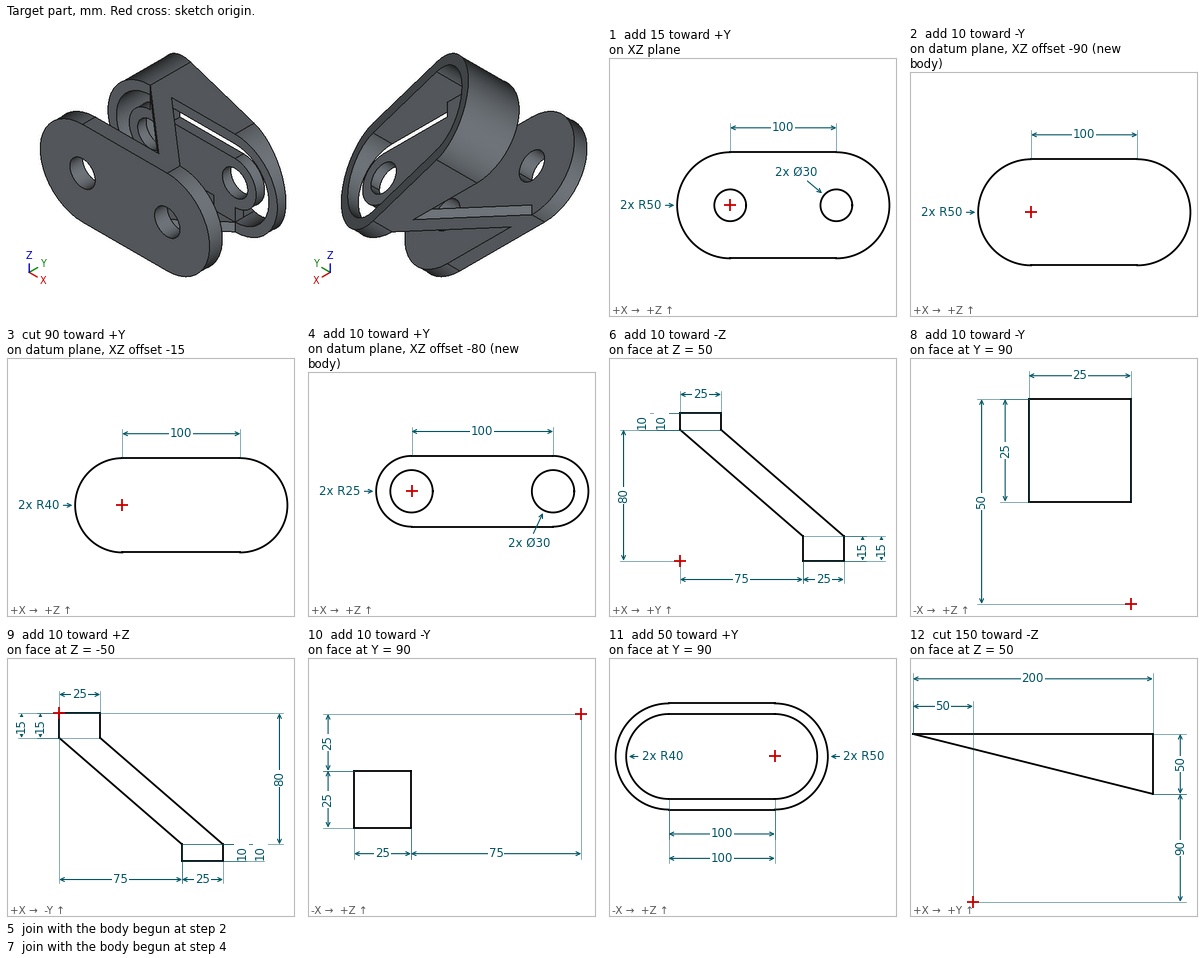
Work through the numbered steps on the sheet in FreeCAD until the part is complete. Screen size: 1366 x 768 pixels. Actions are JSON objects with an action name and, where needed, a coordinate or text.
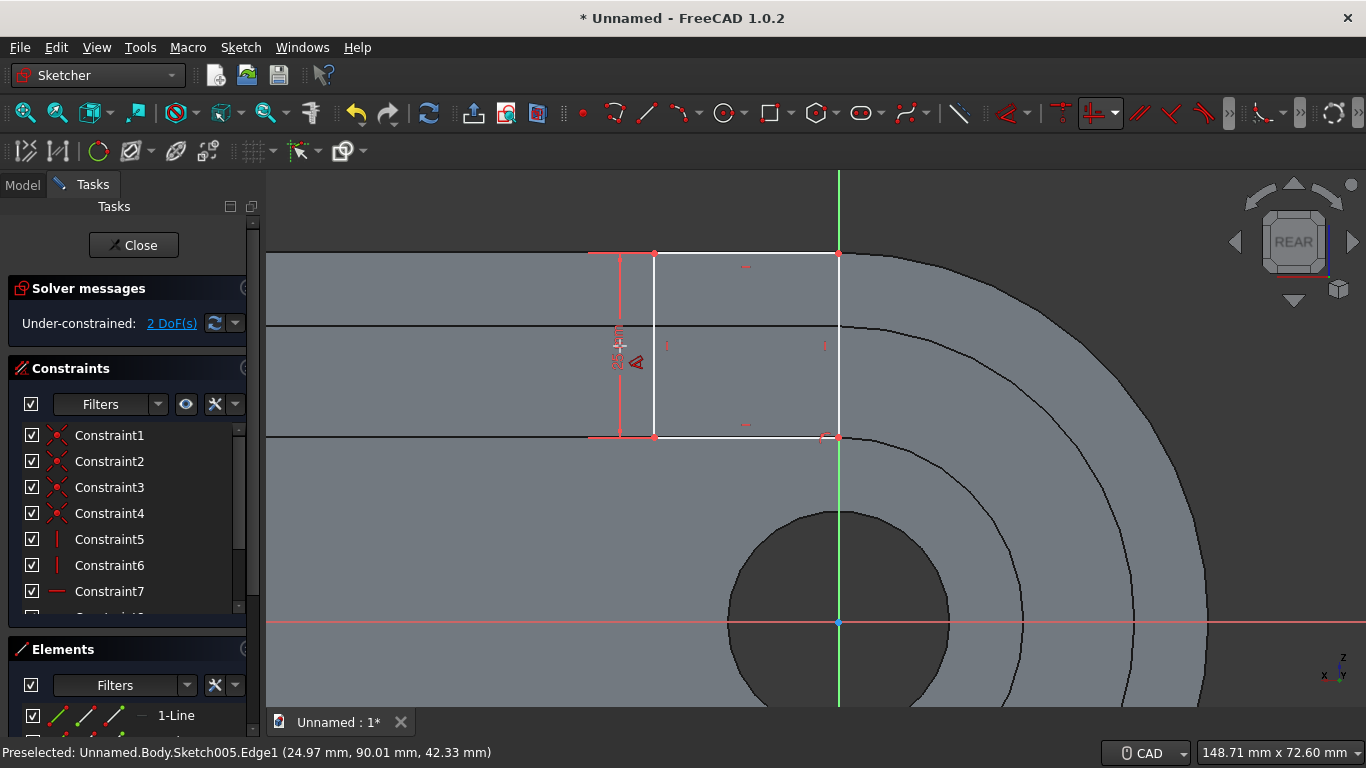
{"action": "left_click", "coordinate": [709, 438]}
{"action": "left_click", "coordinate": [746, 472]}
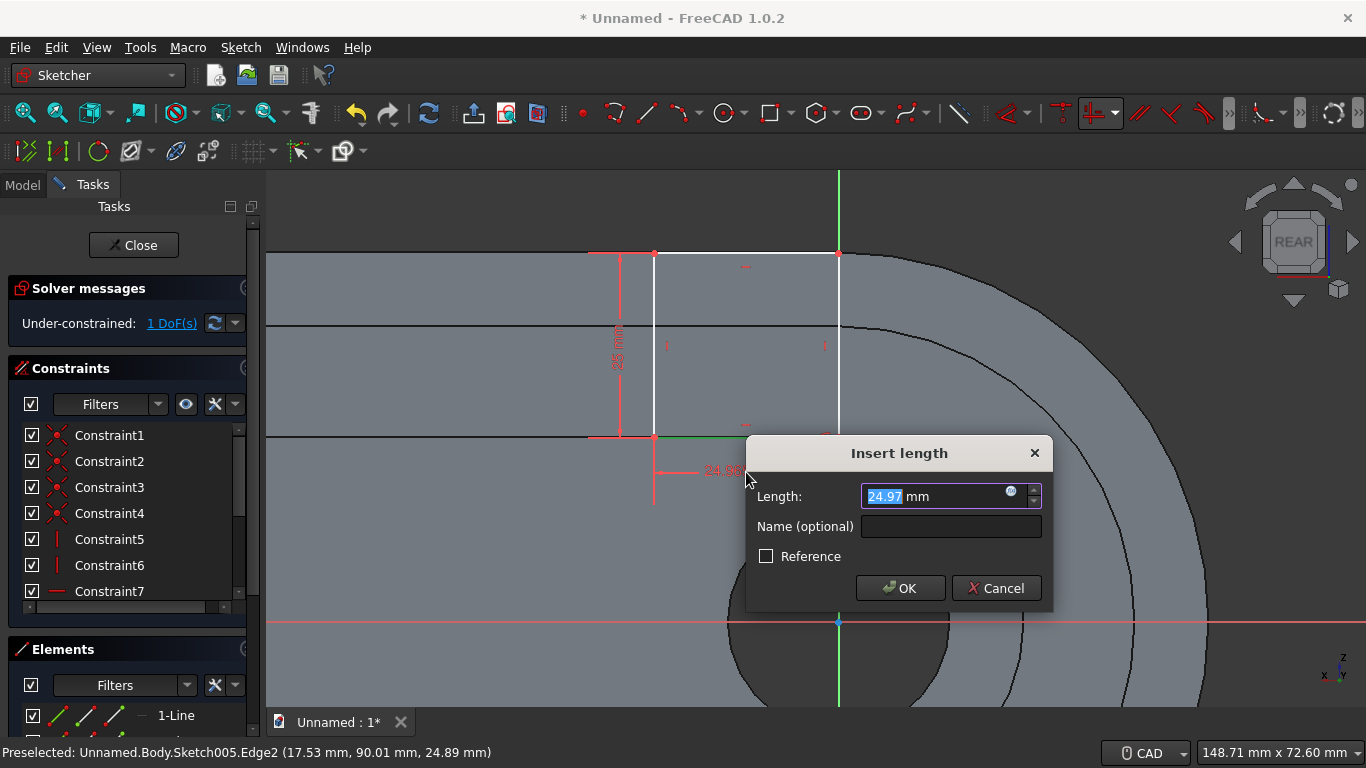
{"action": "type", "text": "25"}
{"action": "key", "text": "Return"}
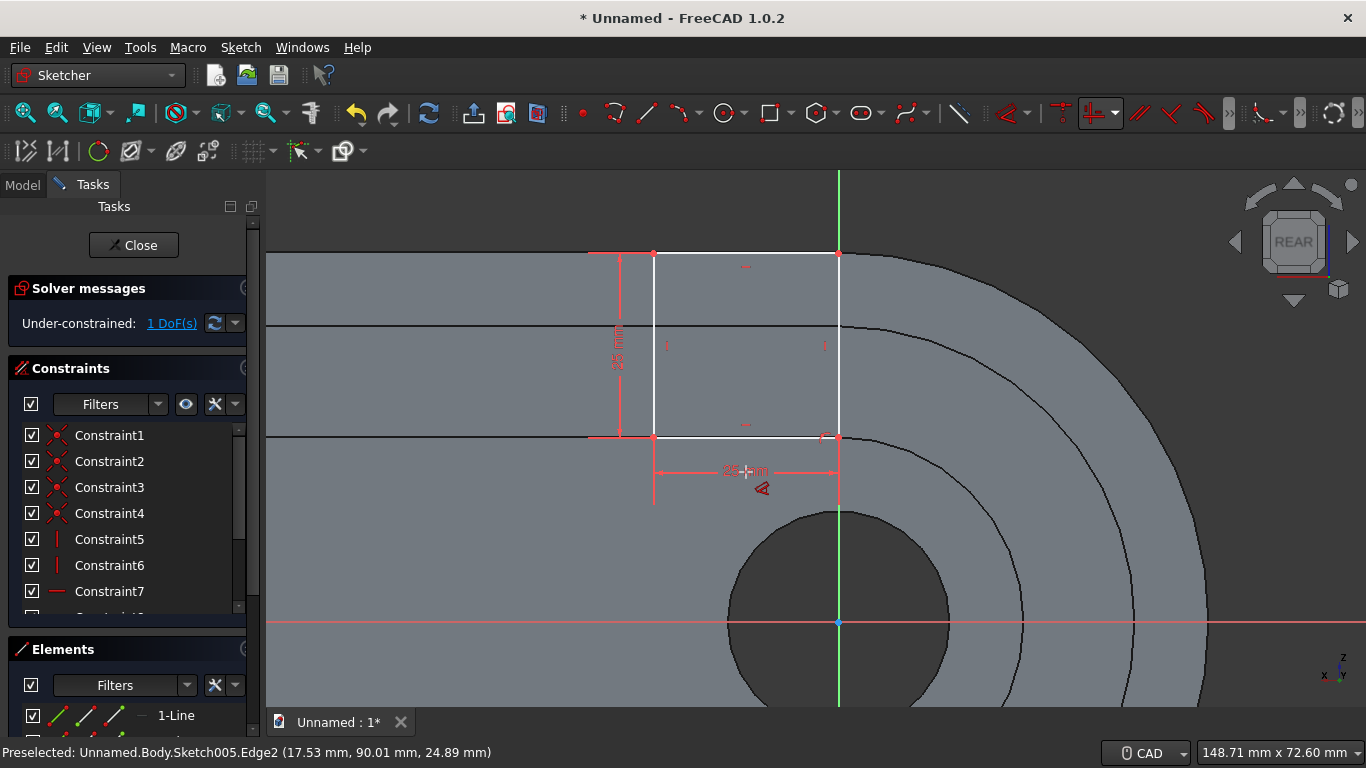
{"action": "left_click", "coordinate": [654, 253]}
{"action": "left_click", "coordinate": [873, 438]}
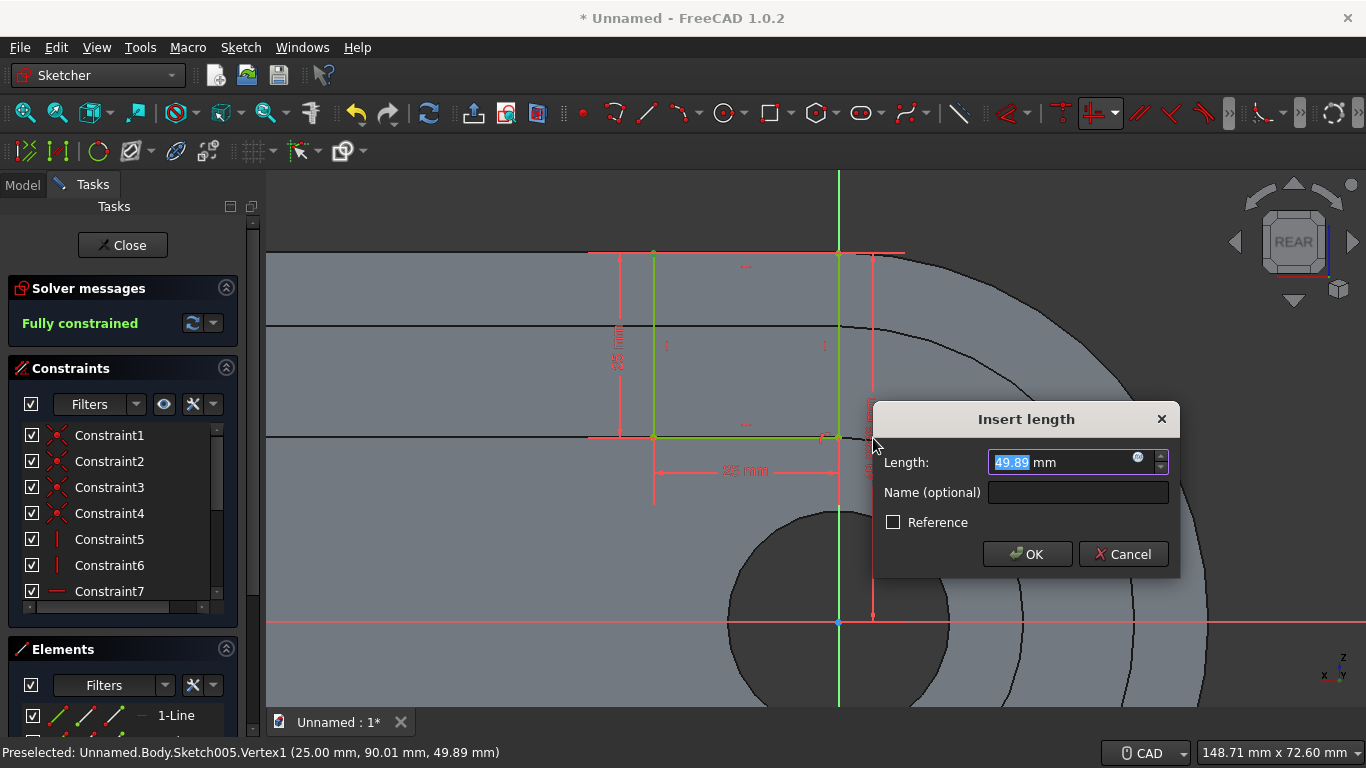
{"action": "type", "text": "50"}
{"action": "key", "text": "Return"}
{"action": "key", "text": "Escape"}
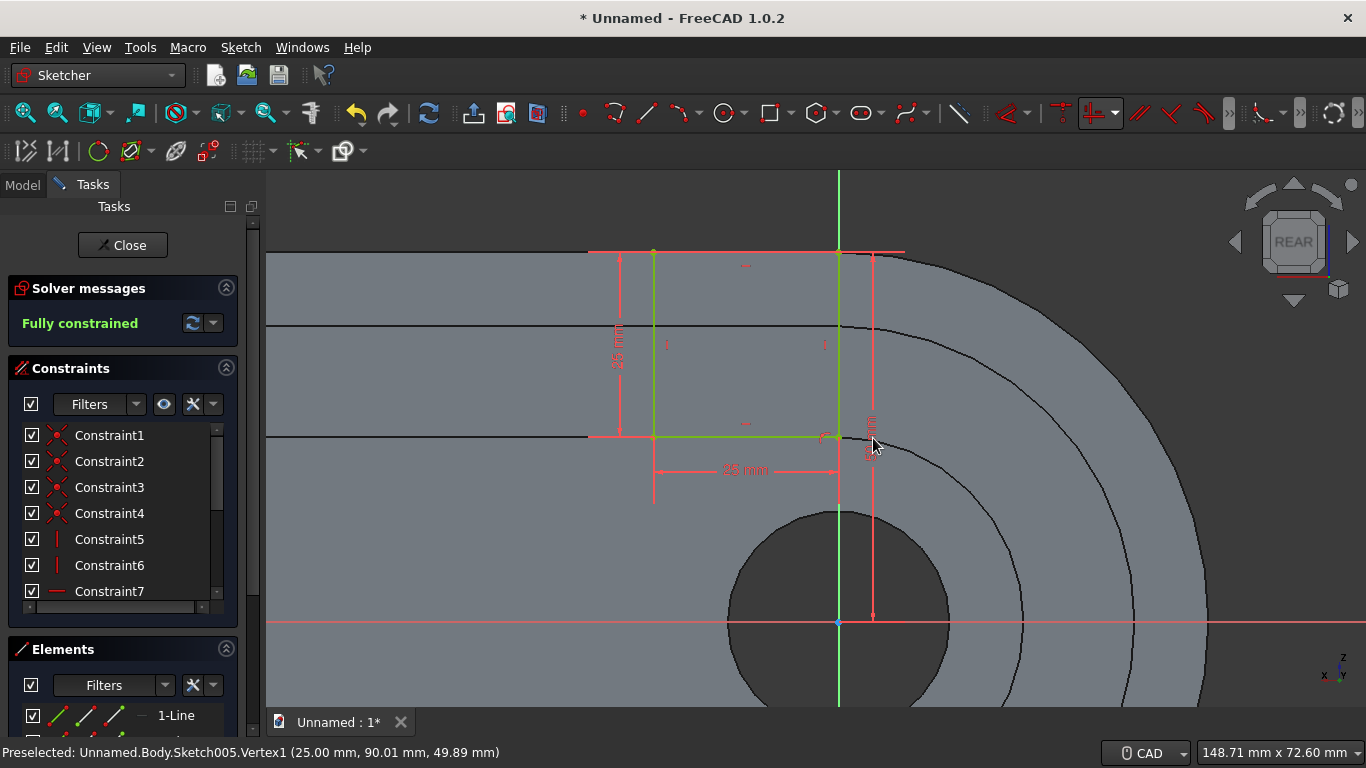
{"action": "left_click", "coordinate": [123, 245]}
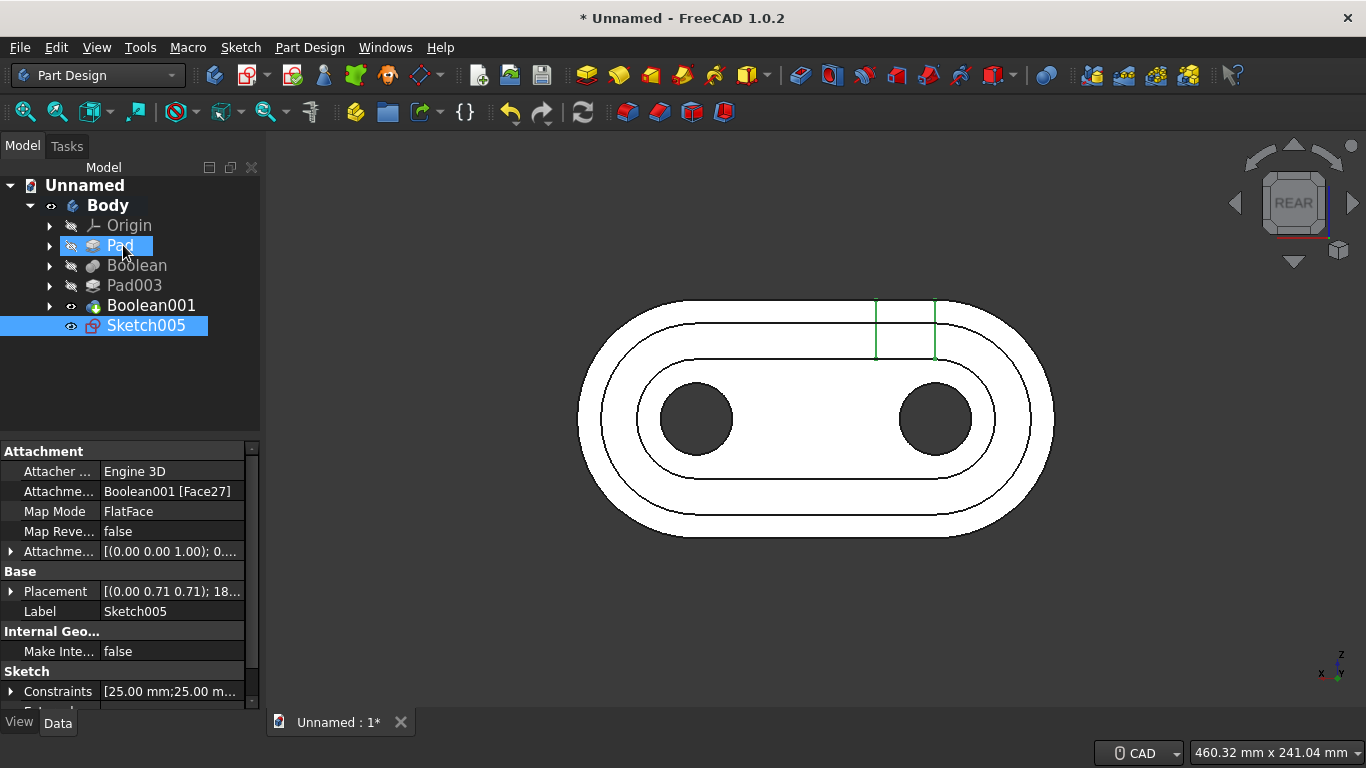
{"action": "left_click", "coordinate": [588, 76]}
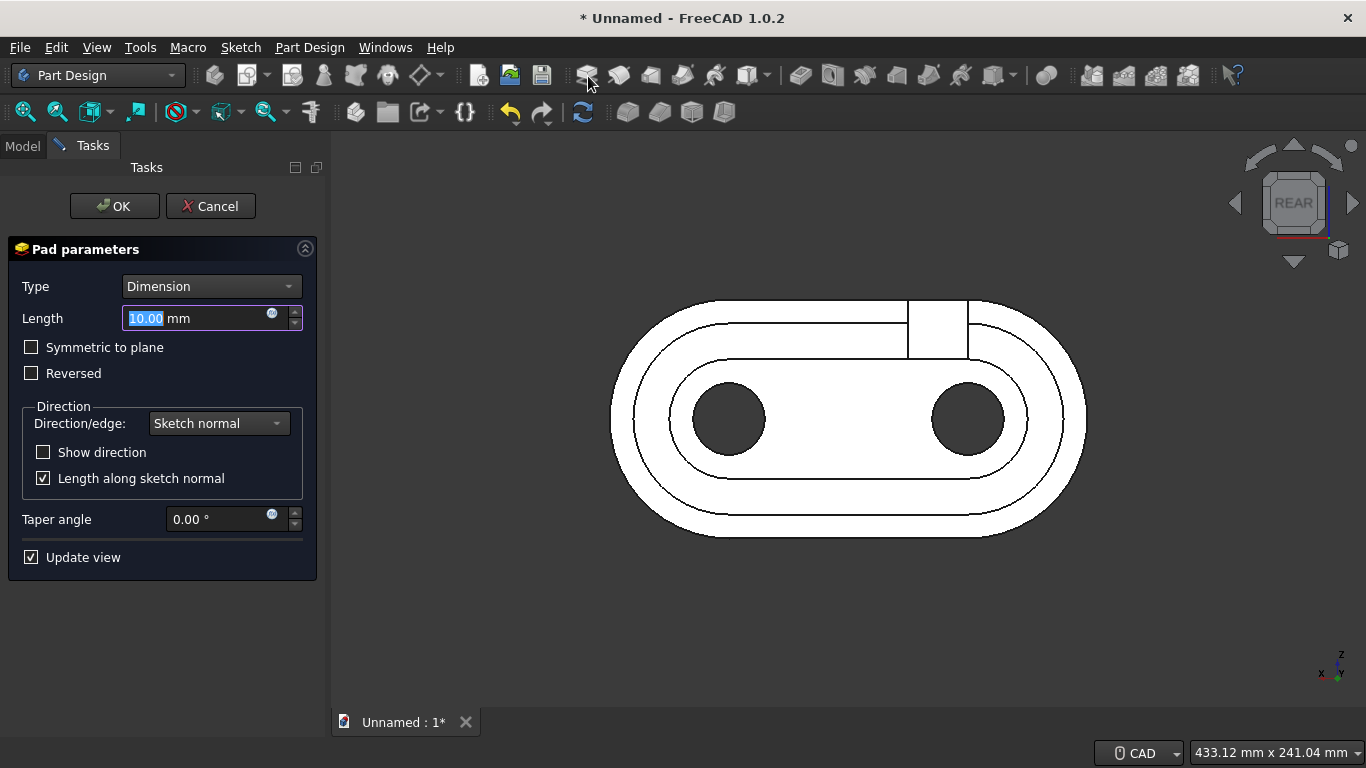
{"action": "type", "text": "10"}
{"action": "key", "text": "Tab"}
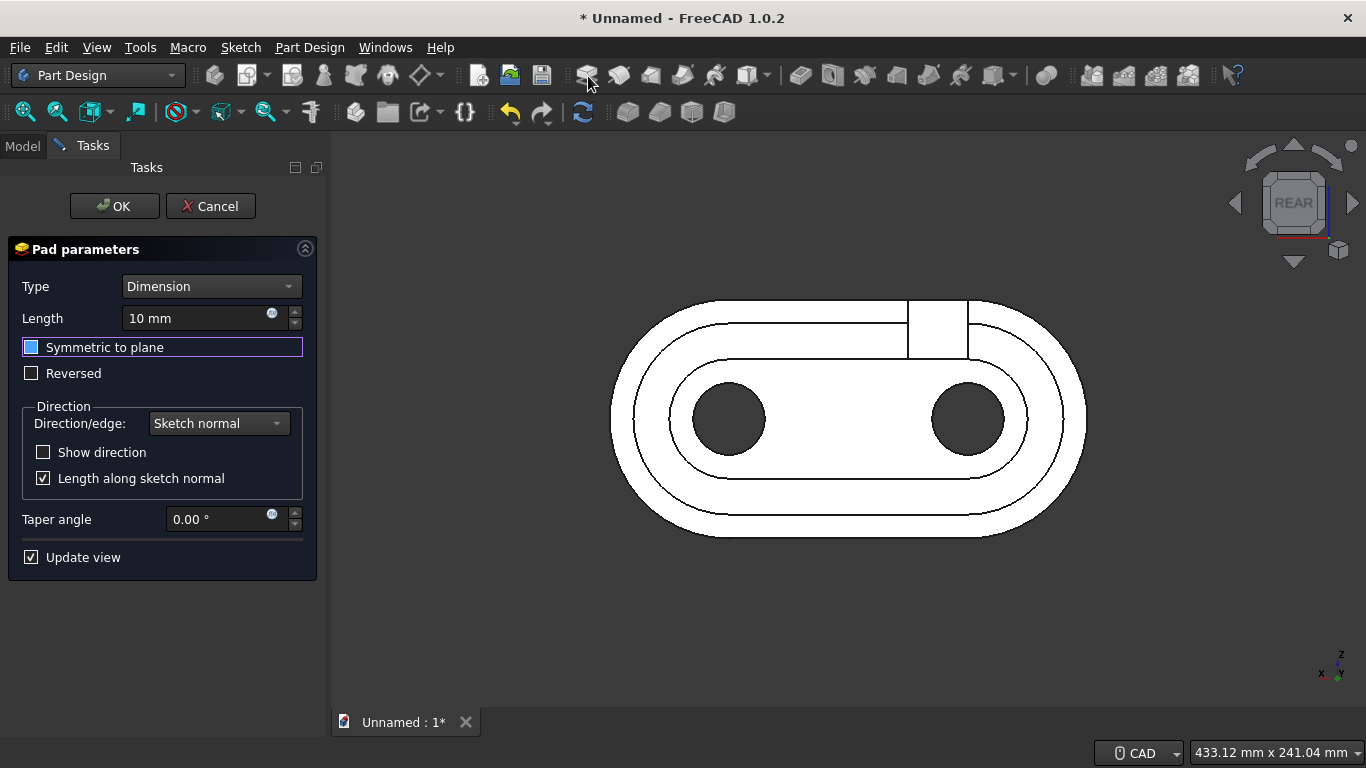
{"action": "left_click", "coordinate": [30, 373]}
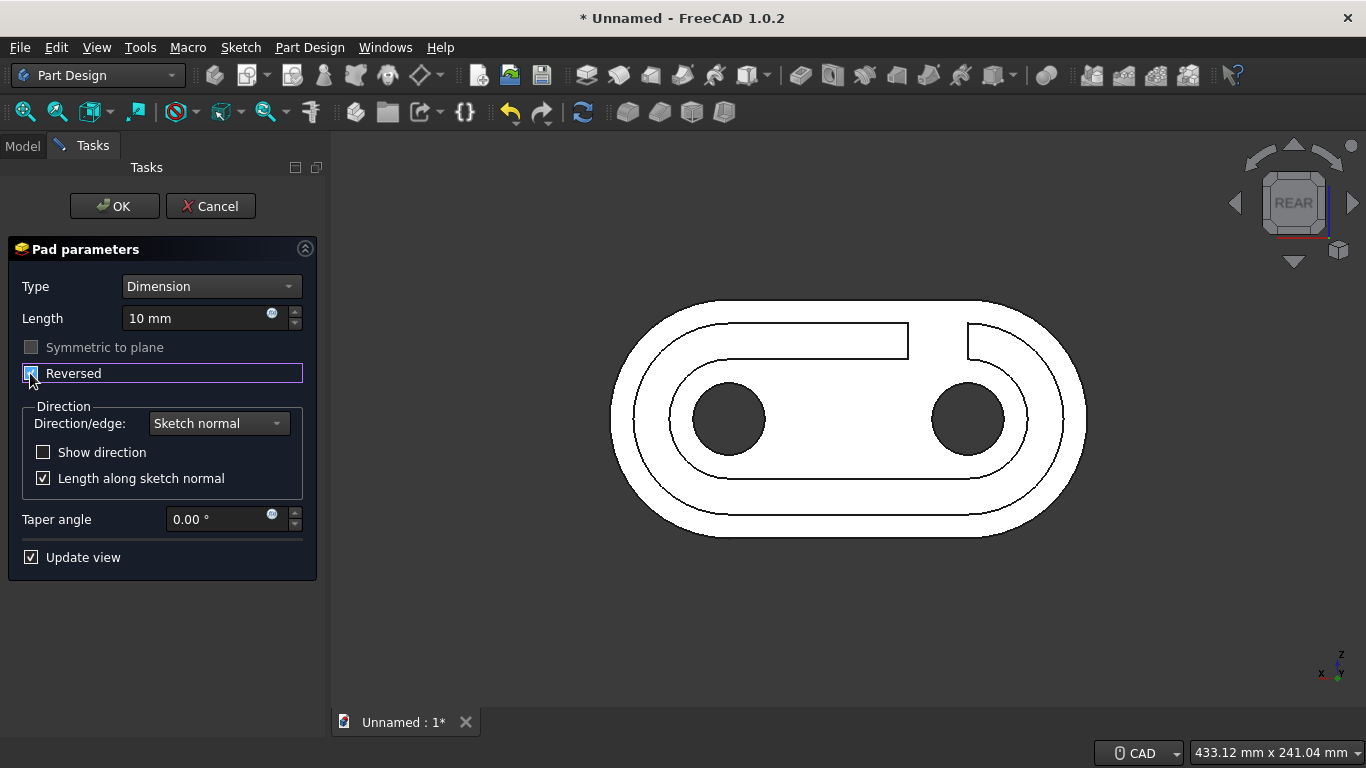
{"action": "left_click", "coordinate": [115, 206]}